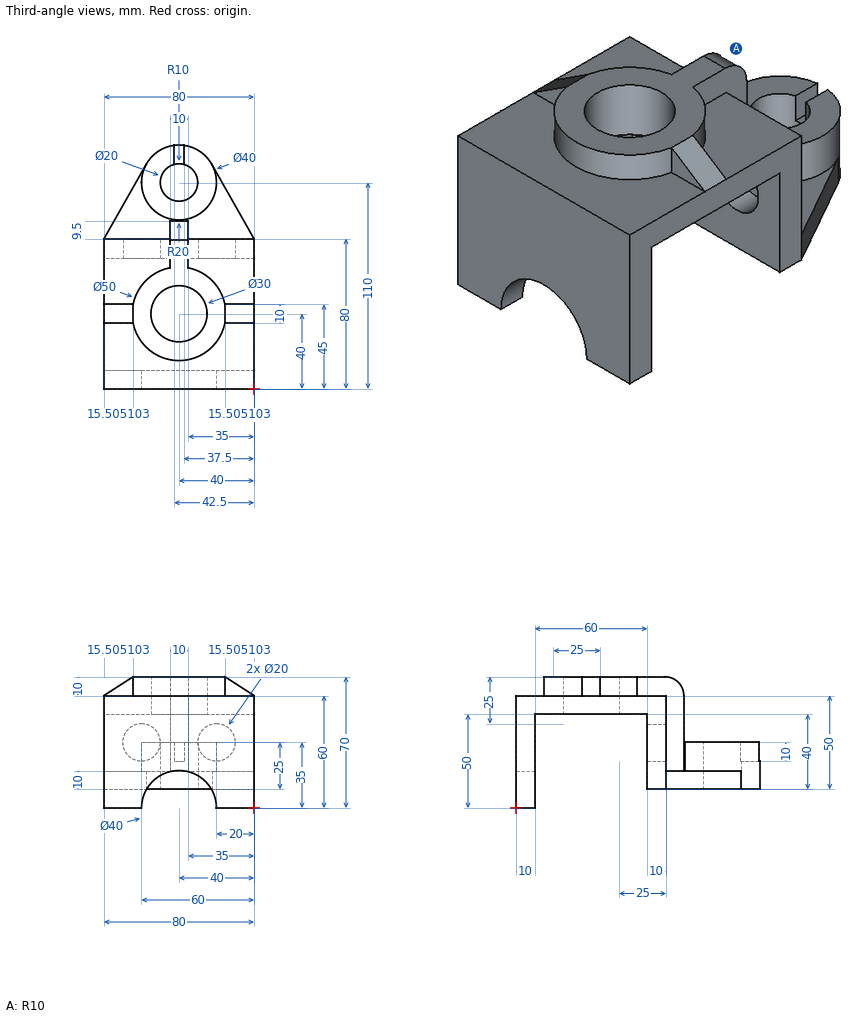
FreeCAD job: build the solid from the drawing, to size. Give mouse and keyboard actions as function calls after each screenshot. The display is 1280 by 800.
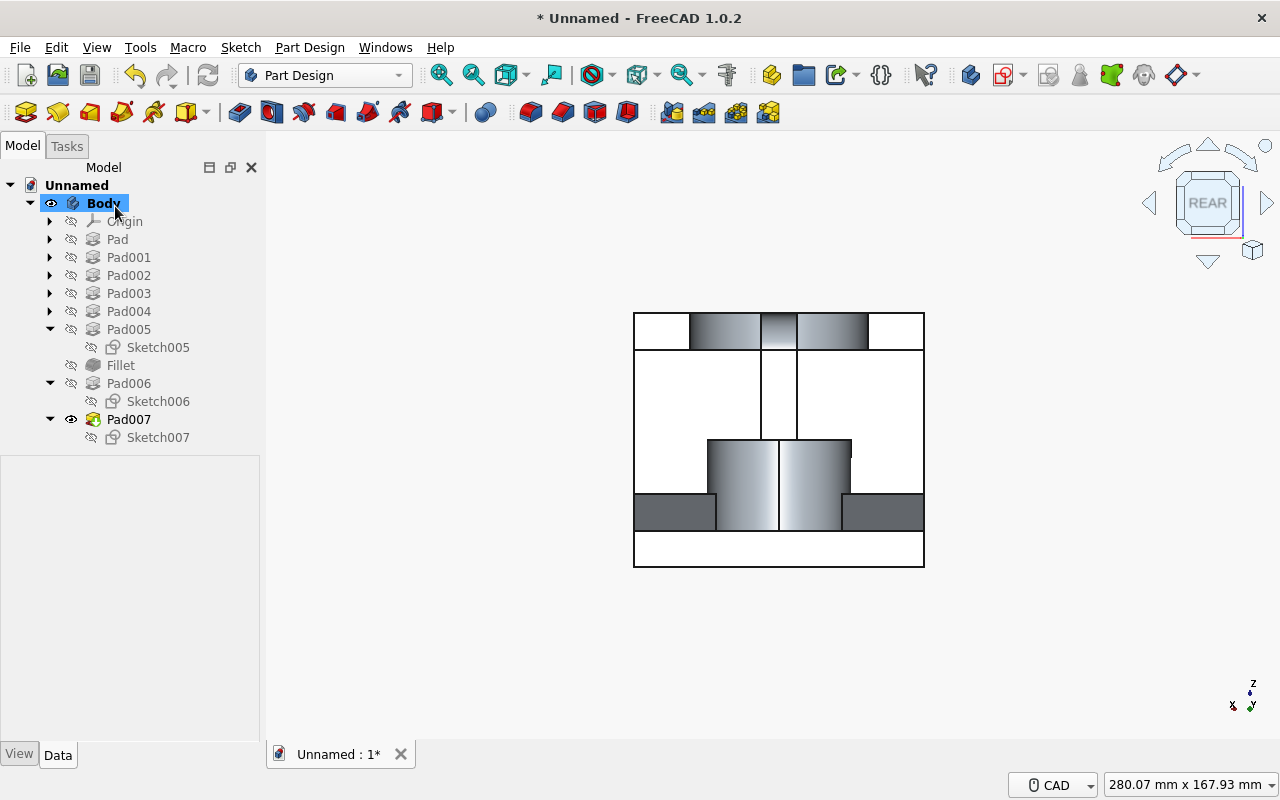
click(442, 76)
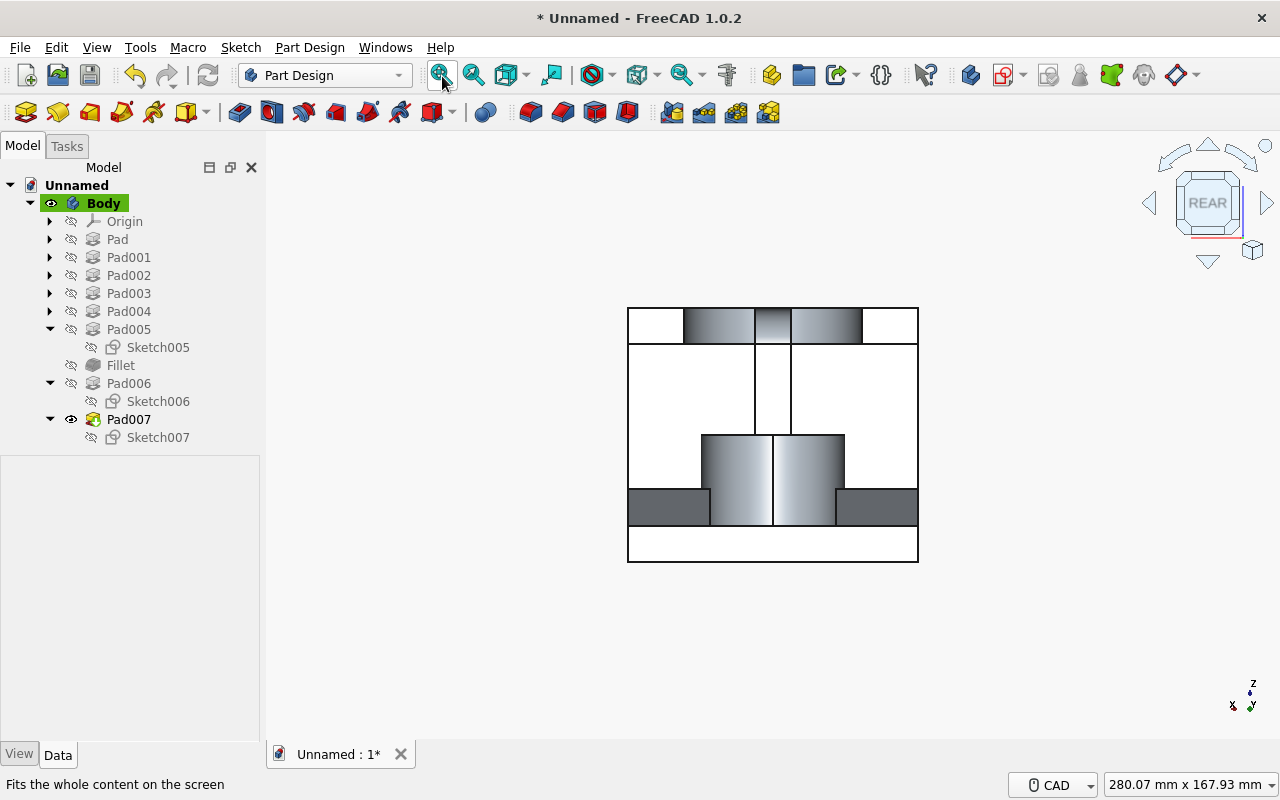
click(664, 325)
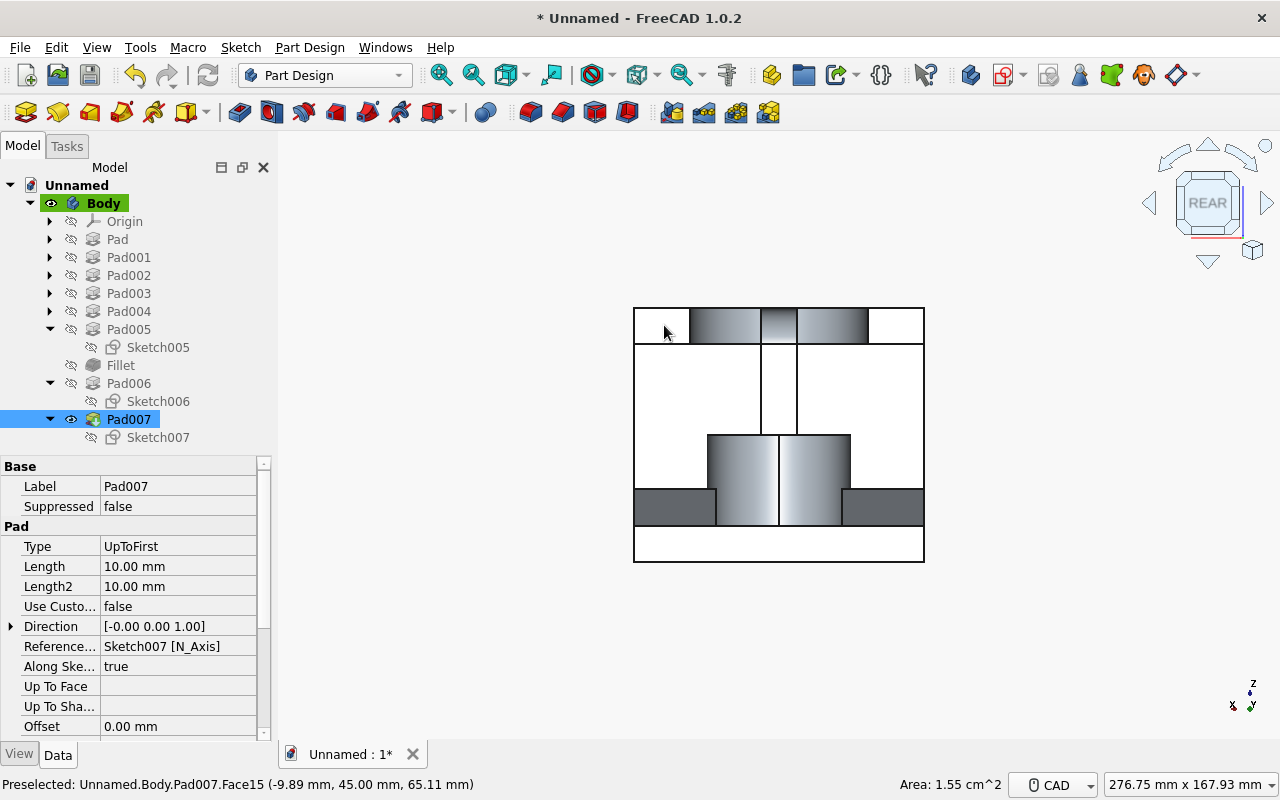
click(1004, 76)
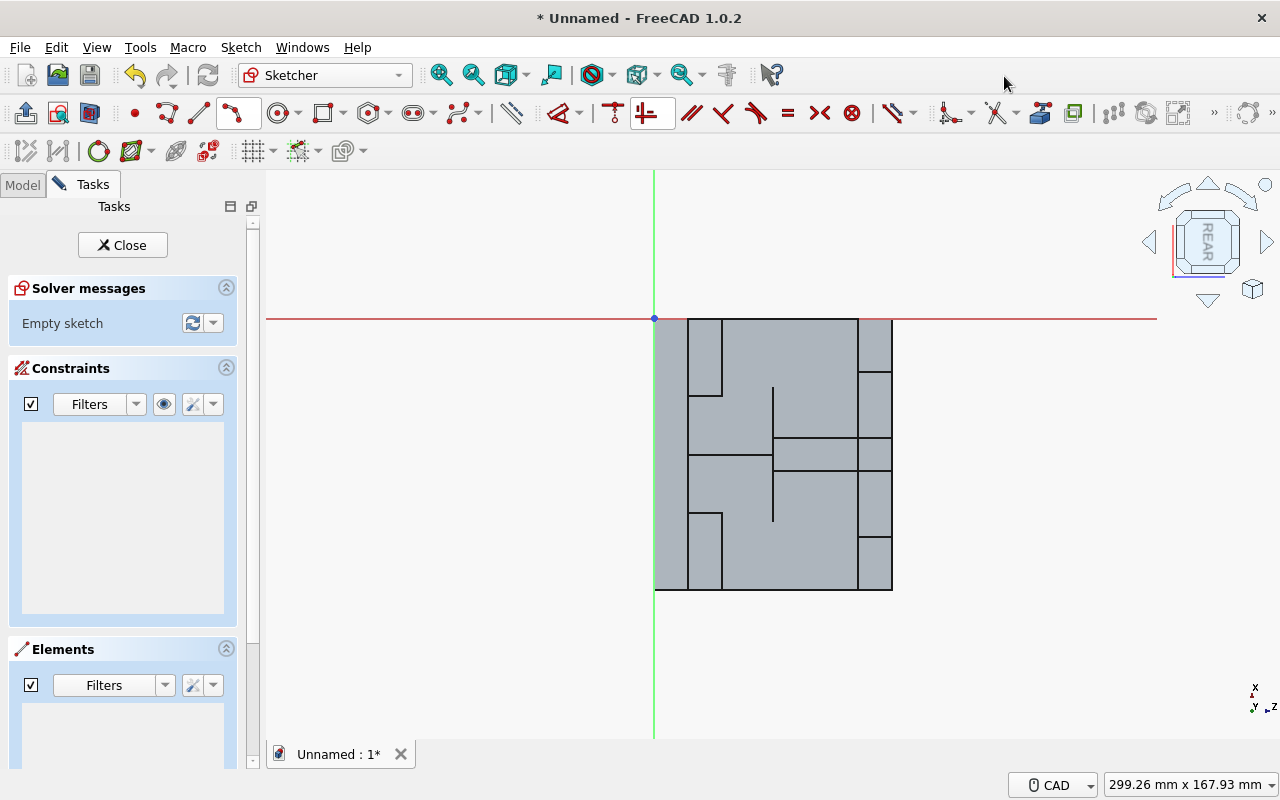
click(168, 114)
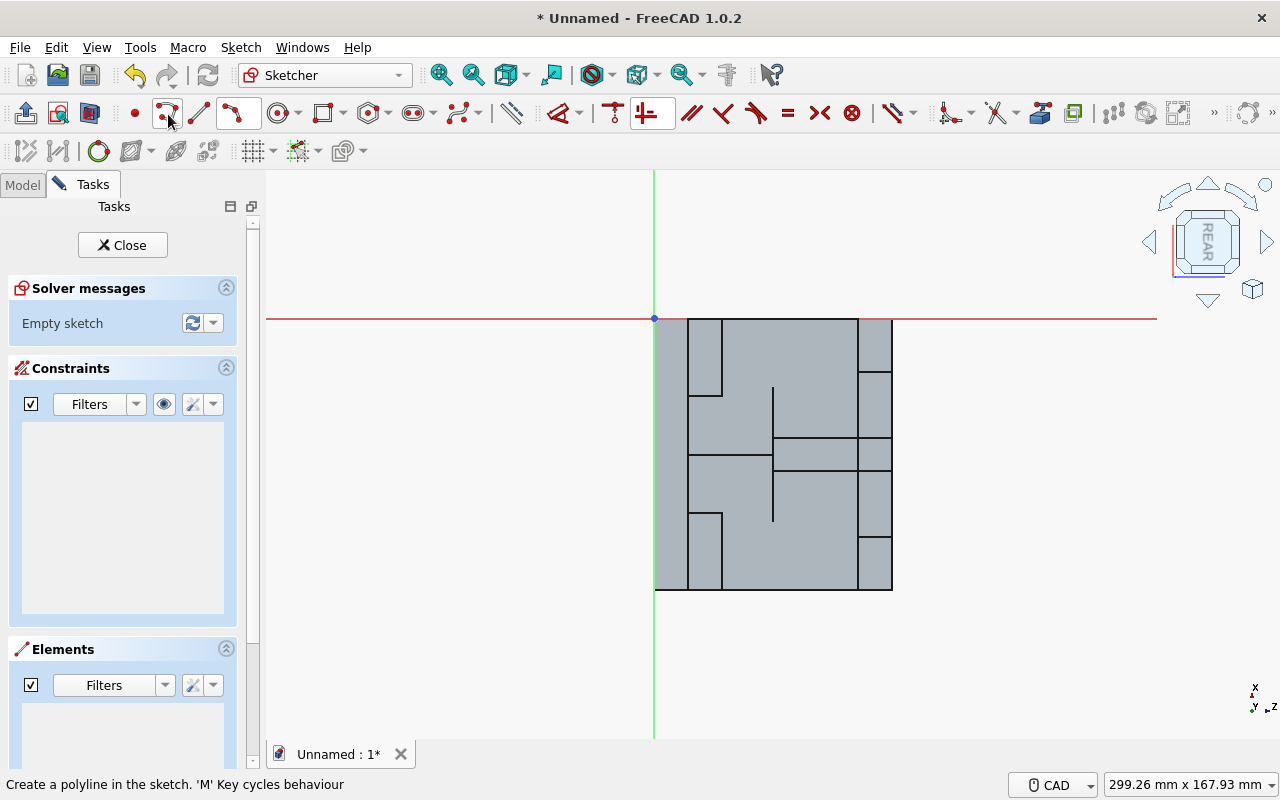
click(858, 319)
click(892, 372)
click(892, 328)
click(858, 319)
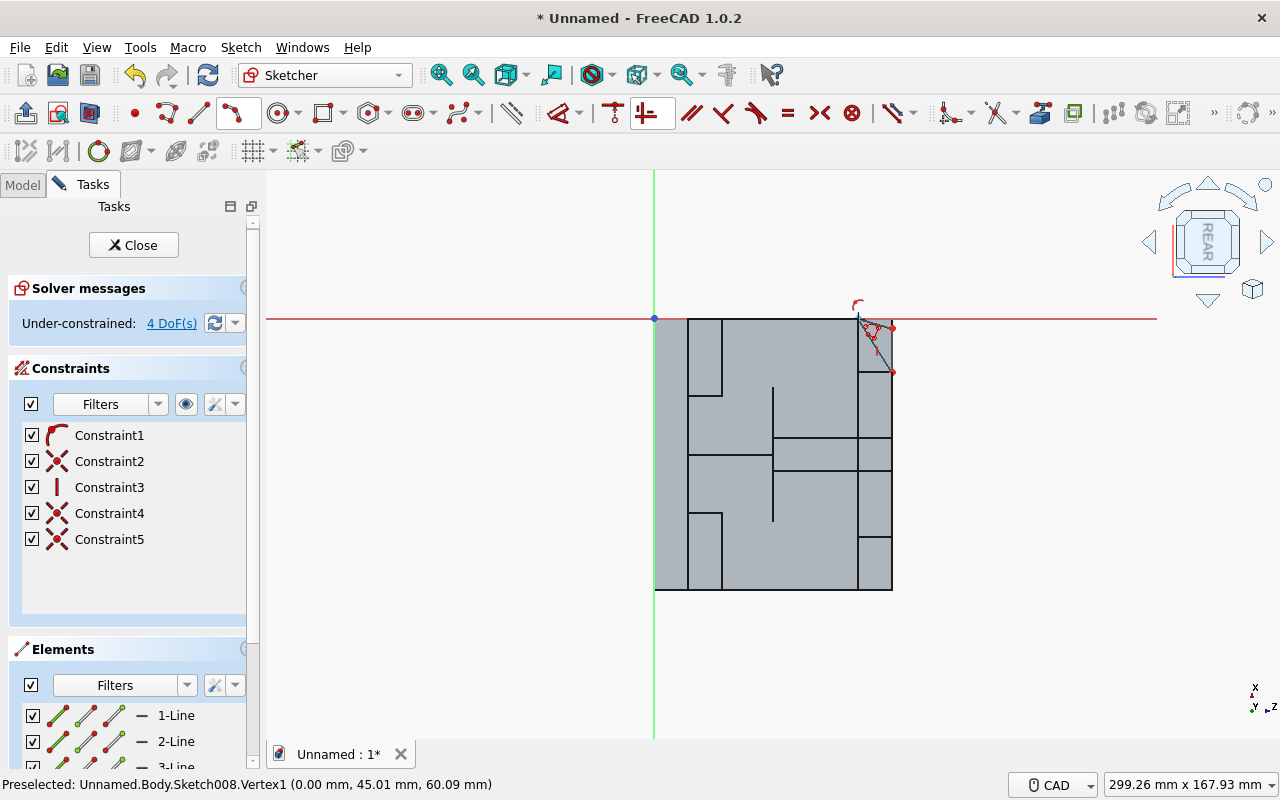
click(892, 537)
click(858, 590)
click(892, 590)
click(892, 538)
key(Escape)
key(Escape)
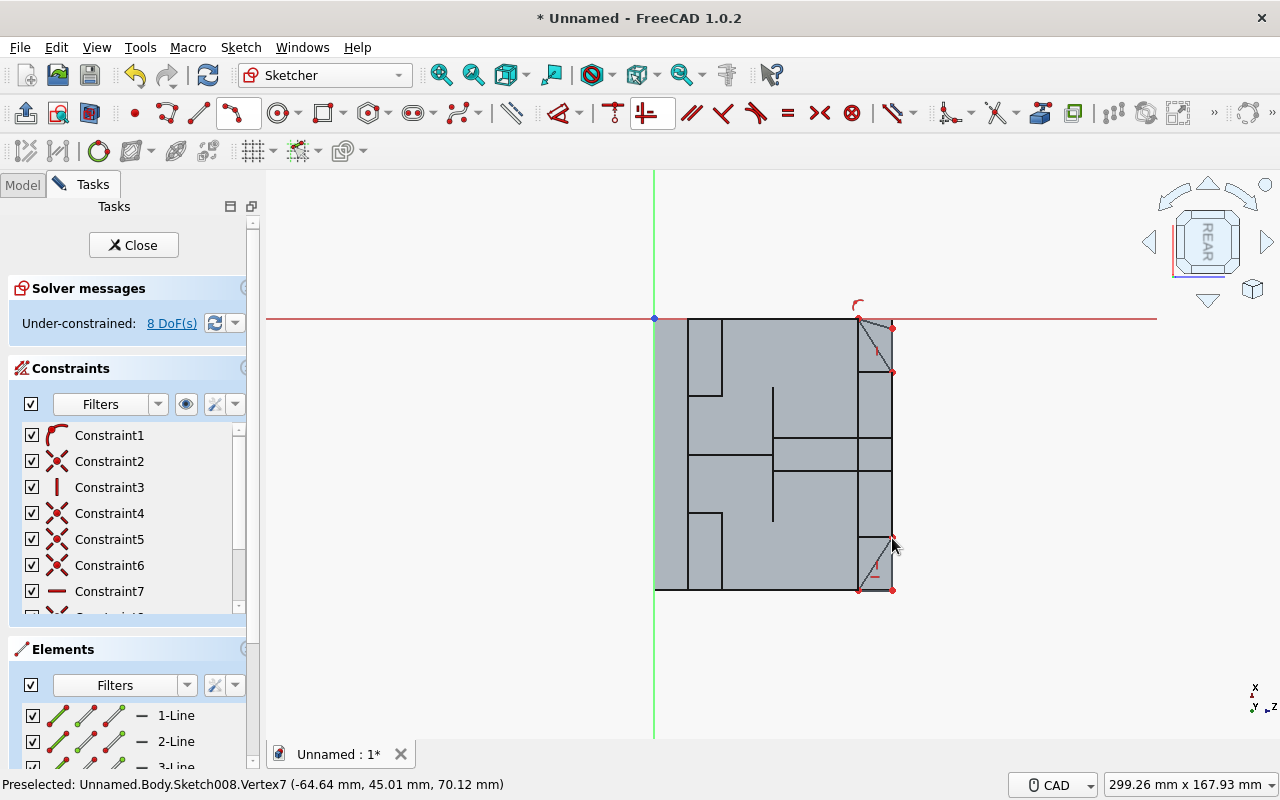
scroll(885, 327, up, 4)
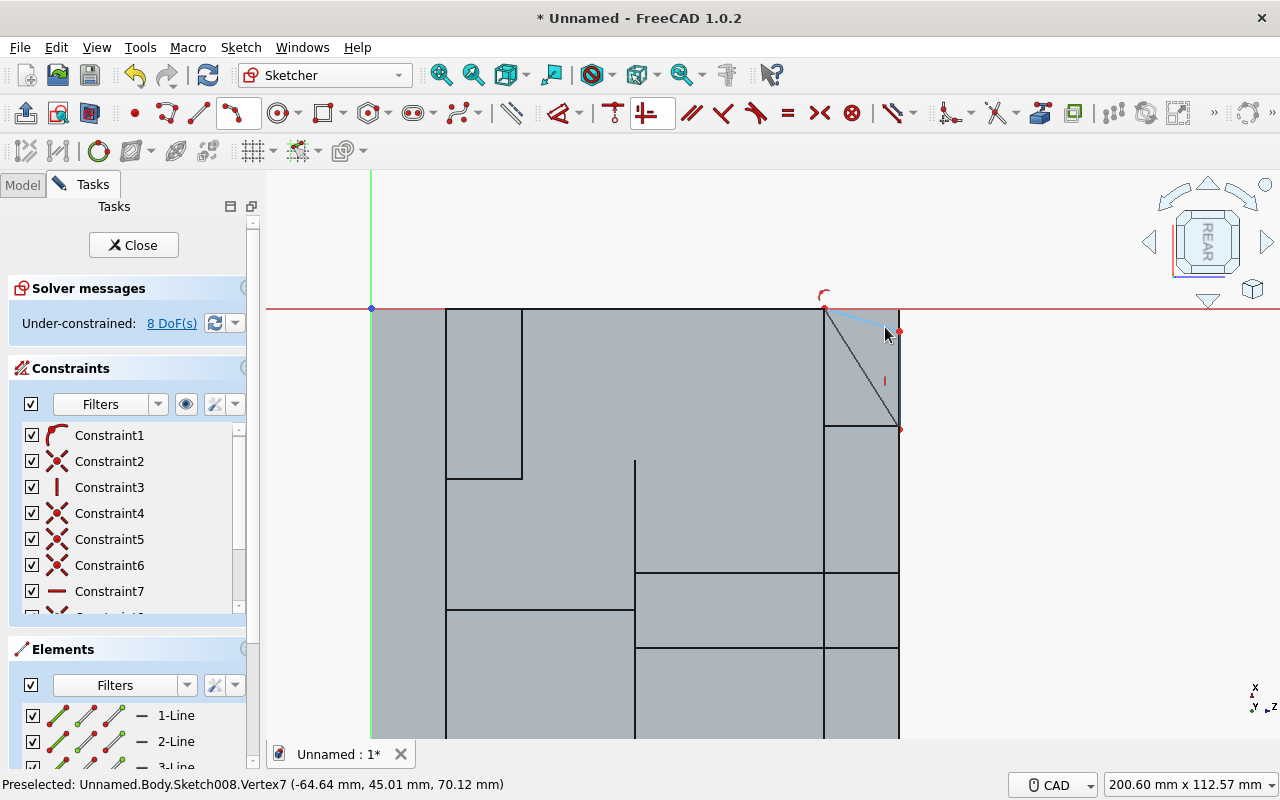
click(885, 327)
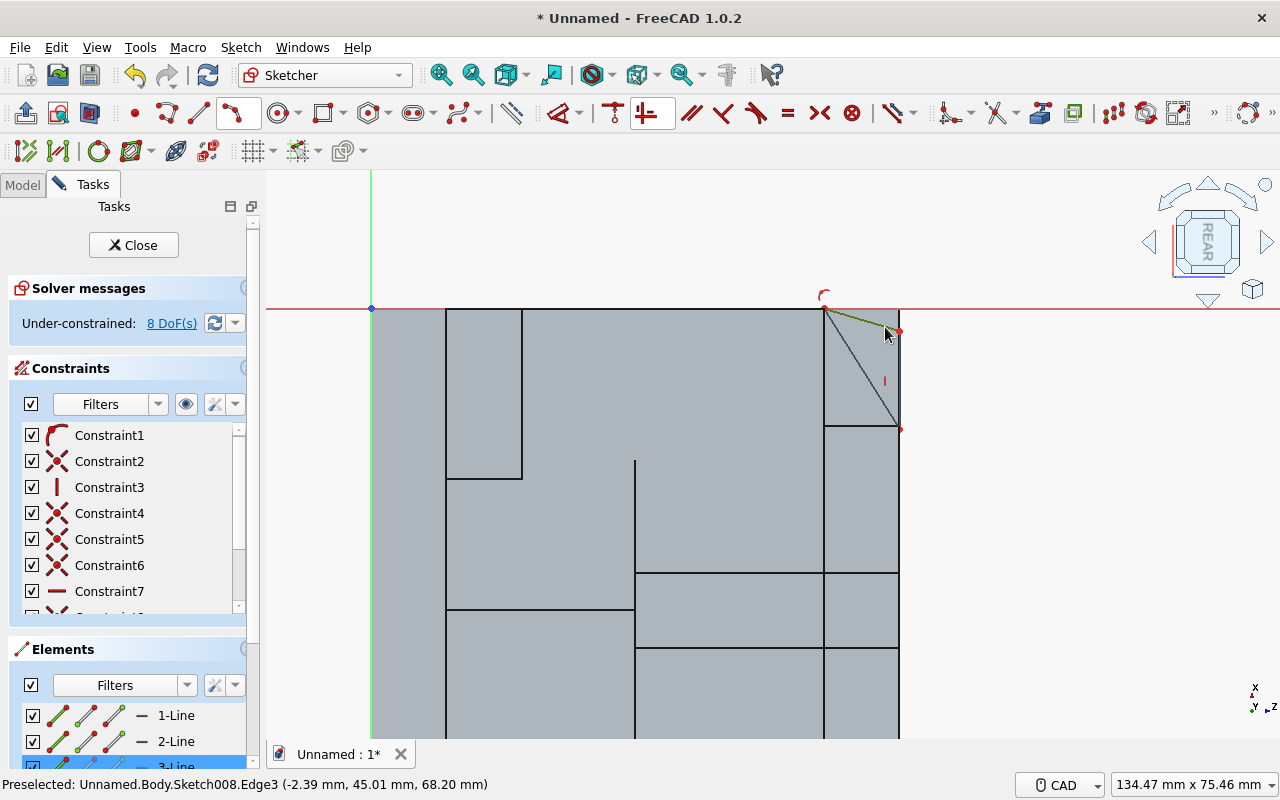
key(h)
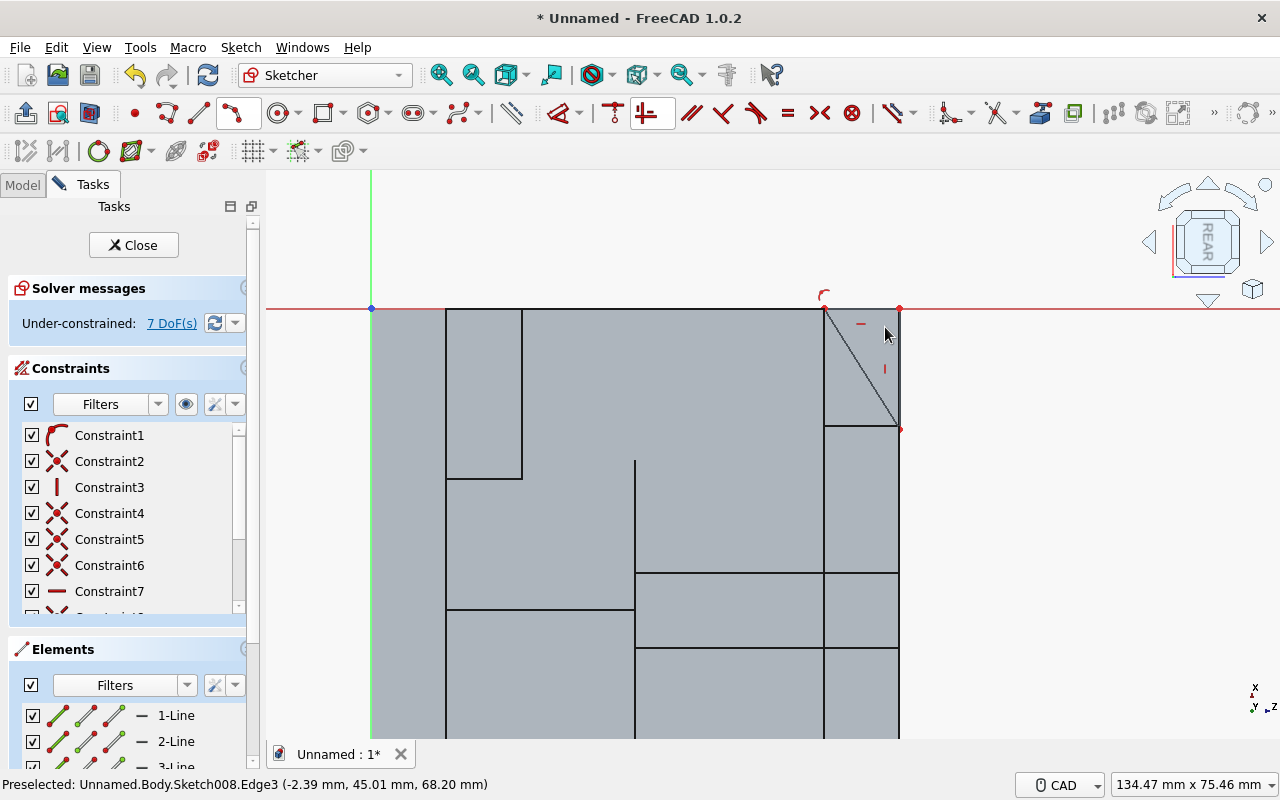
click(558, 114)